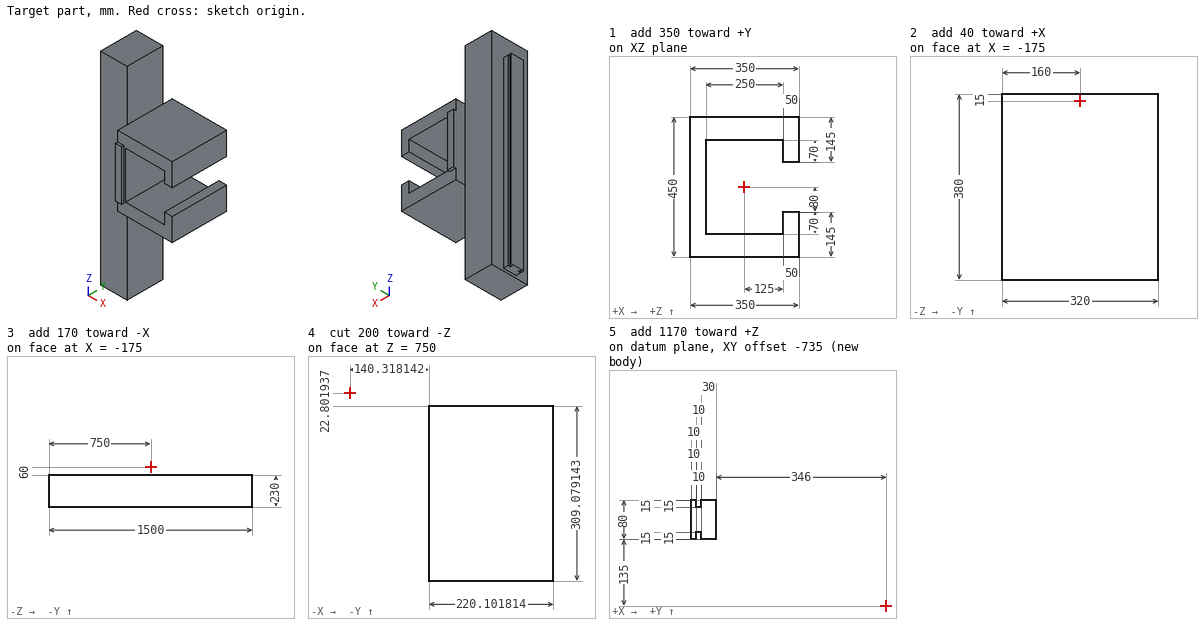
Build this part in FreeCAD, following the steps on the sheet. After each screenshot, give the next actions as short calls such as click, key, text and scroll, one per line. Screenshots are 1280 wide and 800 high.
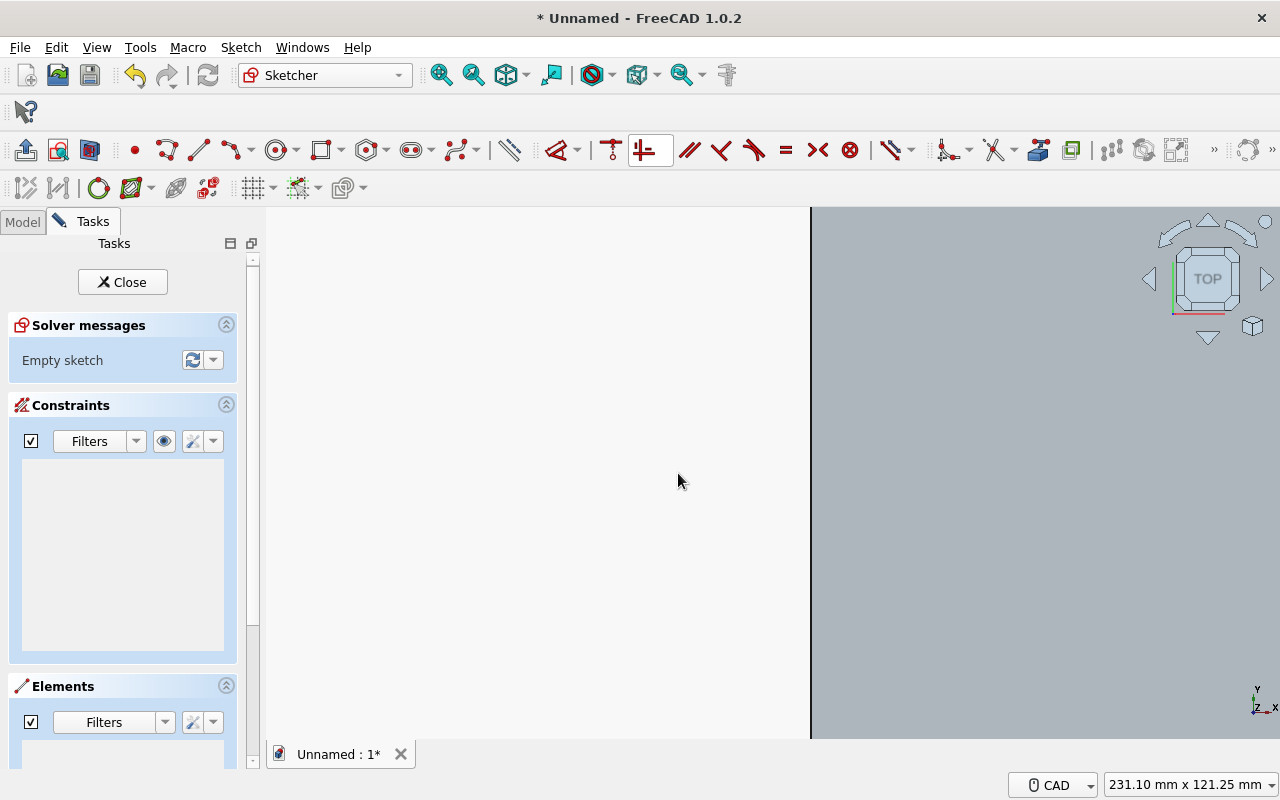
key(g)
key(m)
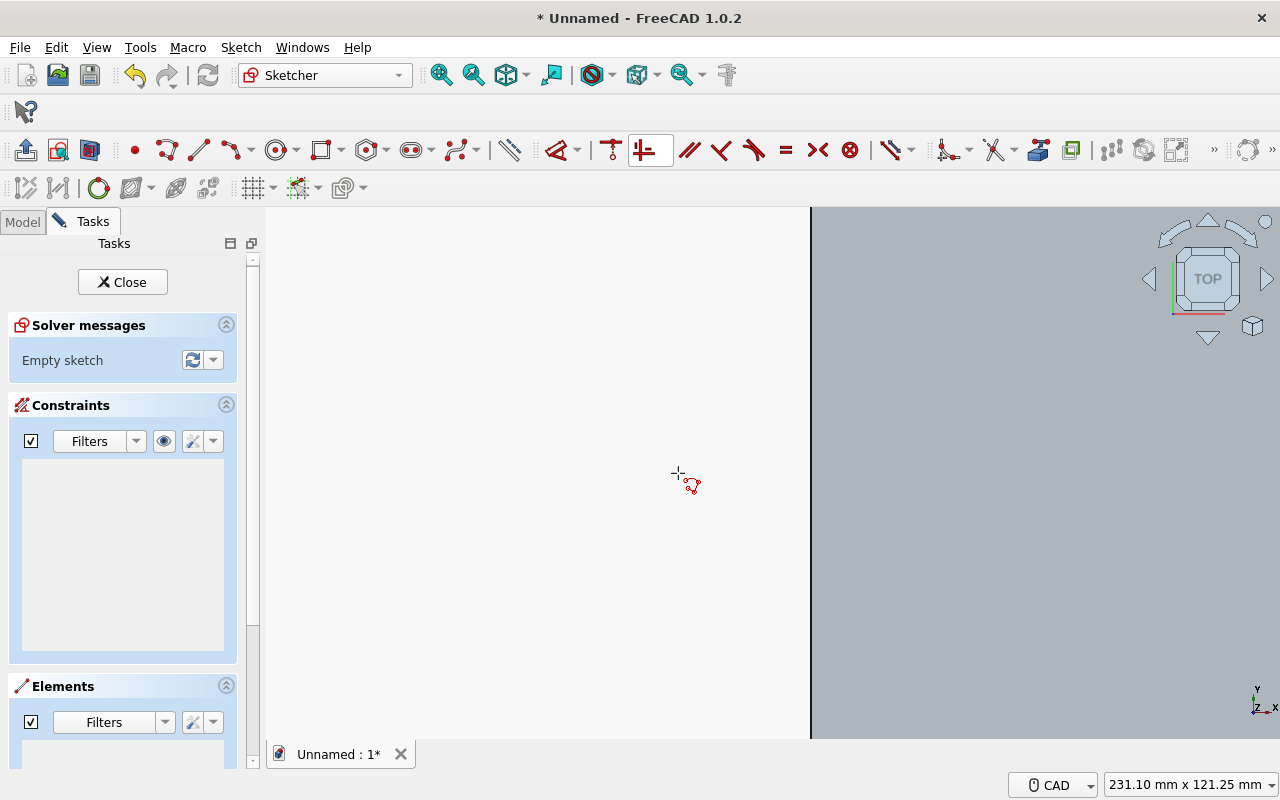
click(807, 642)
click(675, 642)
click(675, 576)
click(631, 576)
click(631, 642)
click(587, 642)
click(587, 291)
click(631, 291)
click(631, 357)
click(675, 357)
click(675, 291)
click(807, 291)
click(807, 643)
key(Escape)
key(Escape)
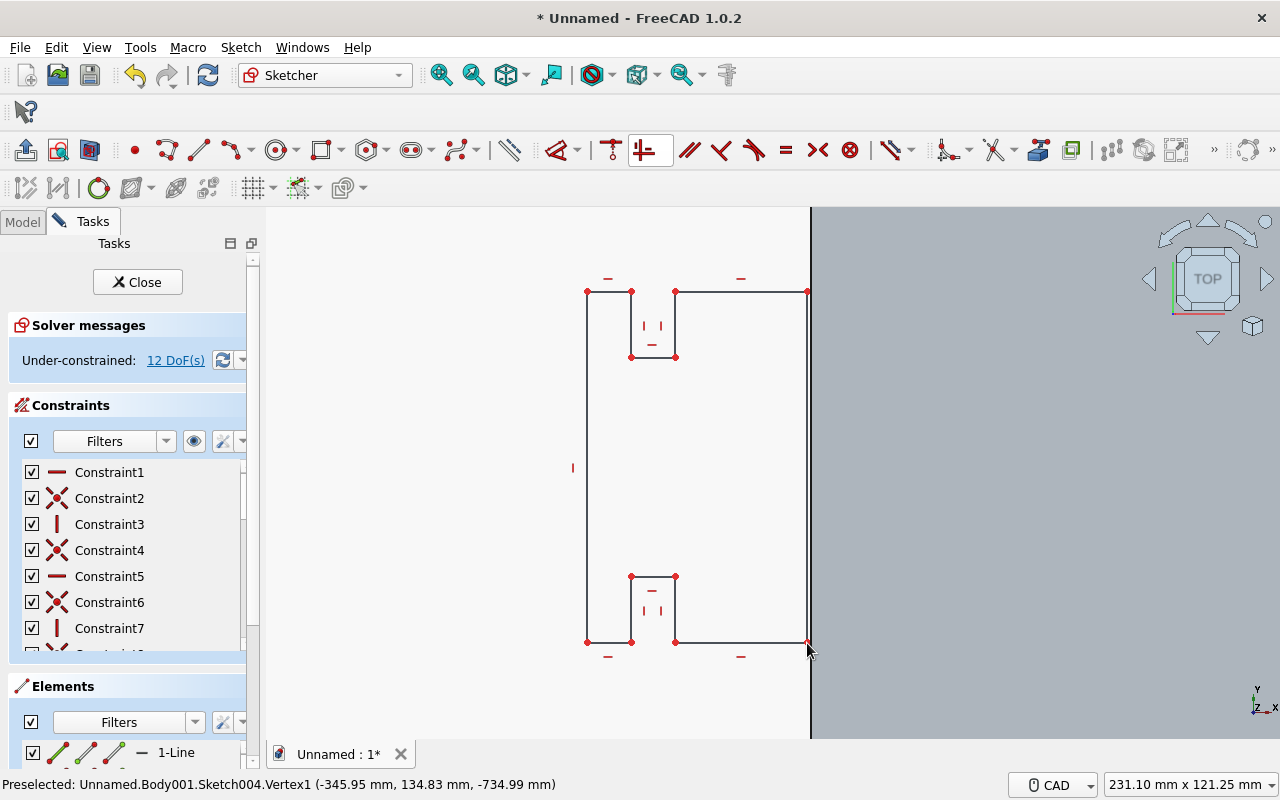
click(556, 150)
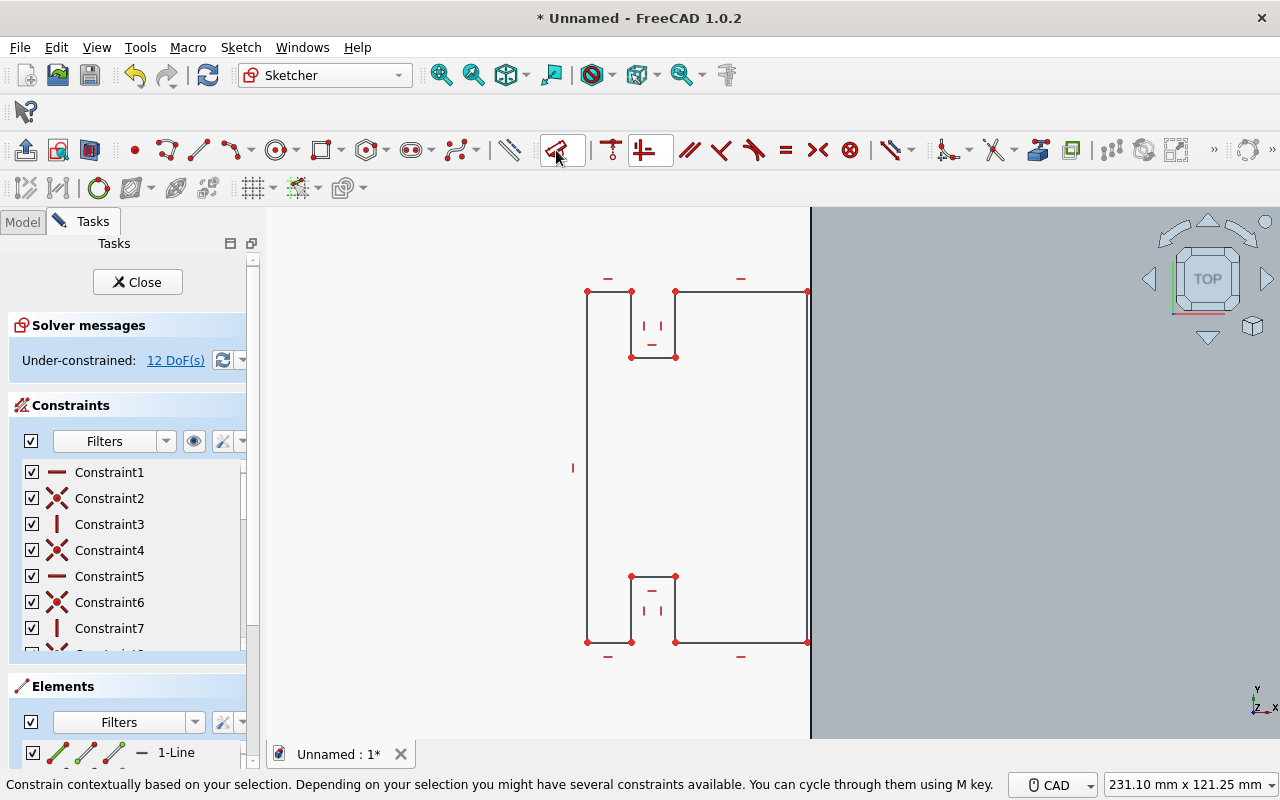
click(767, 643)
click(741, 677)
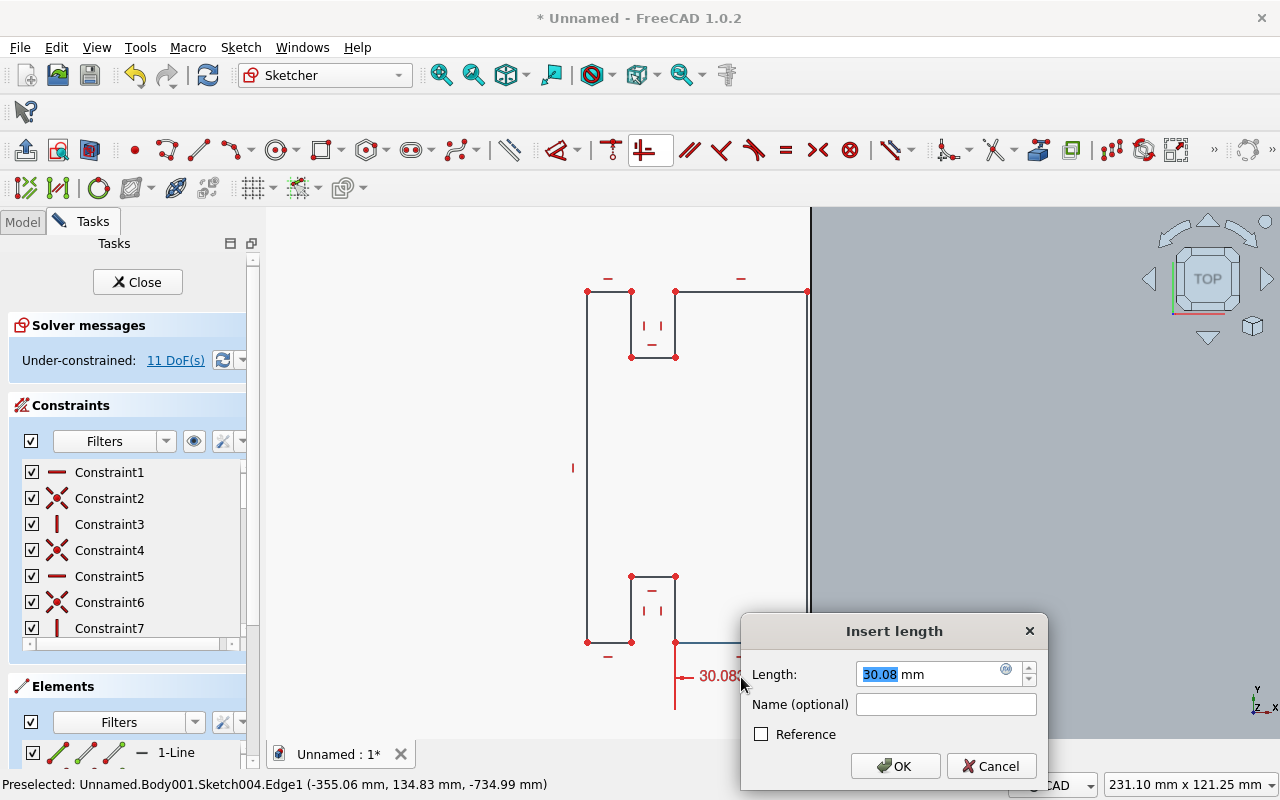
text(30)
key(Return)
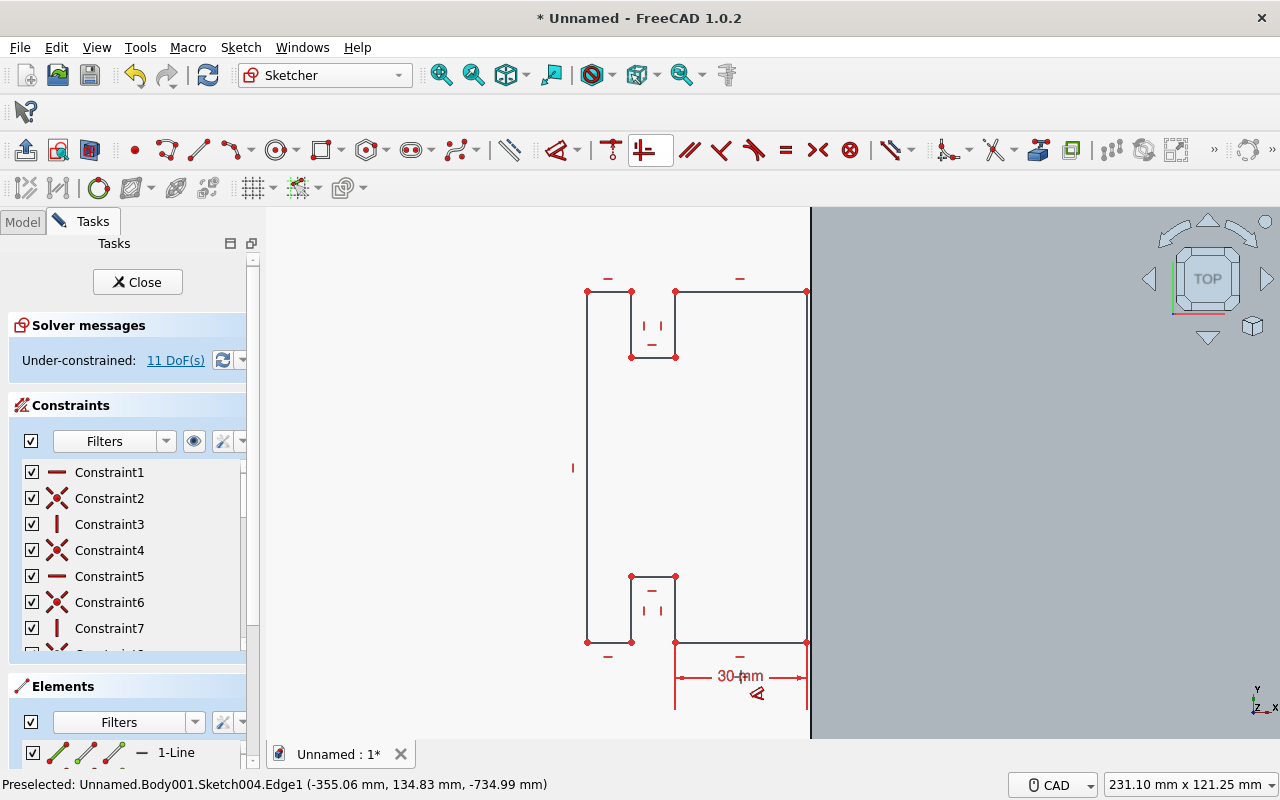
click(675, 623)
click(709, 610)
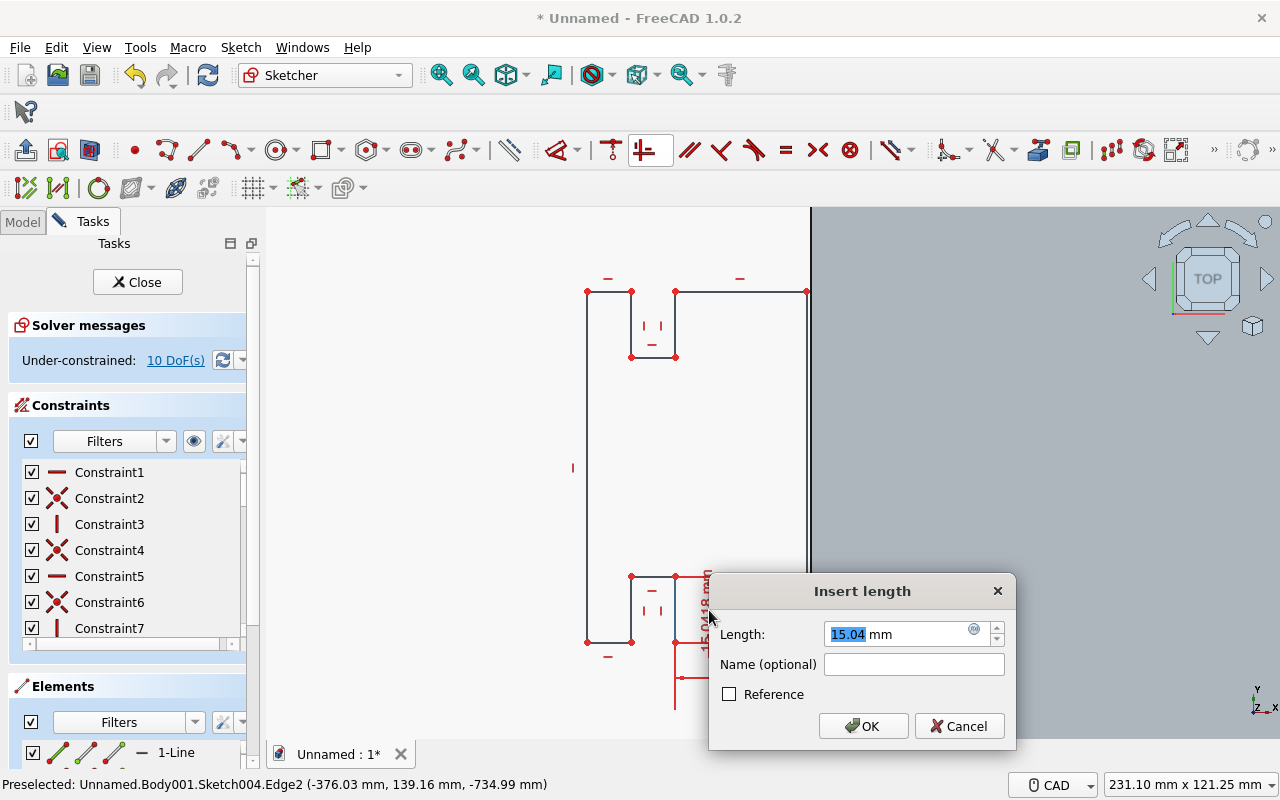
text(15)
key(Return)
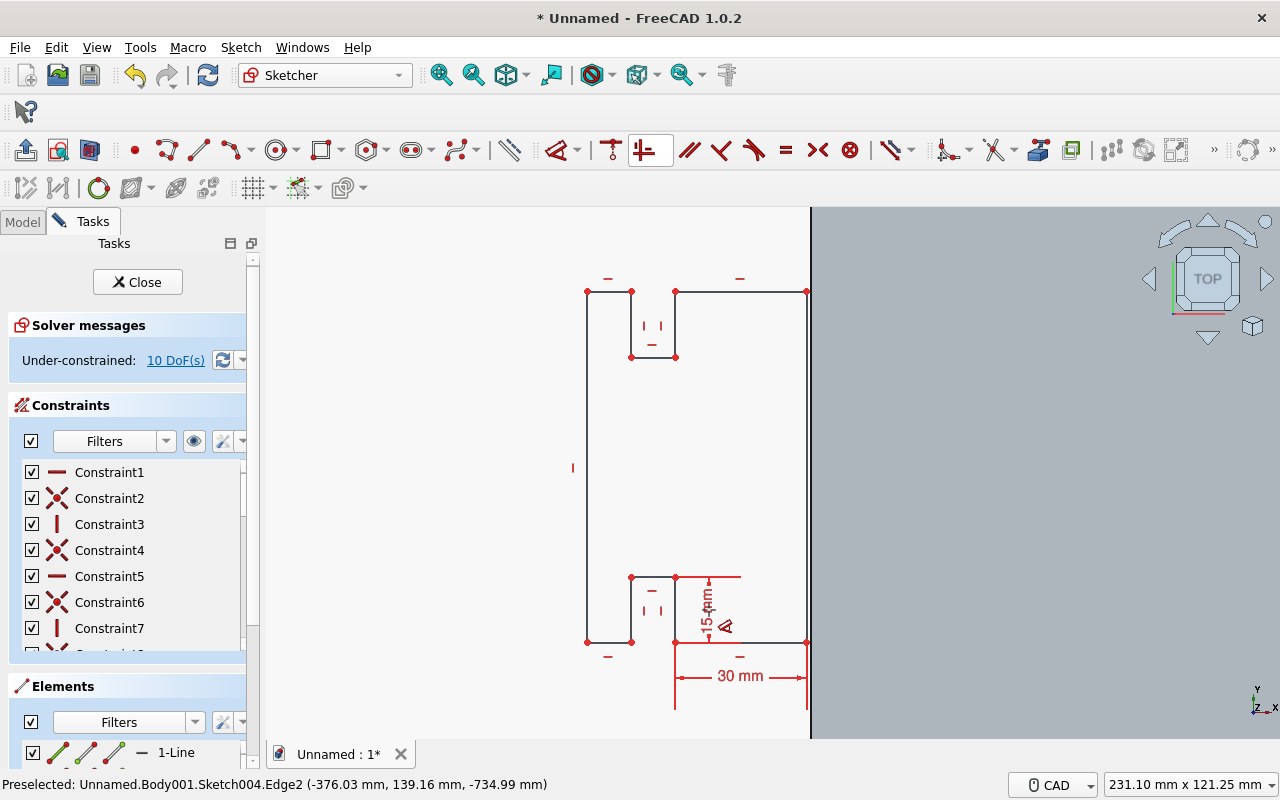
click(662, 577)
click(653, 543)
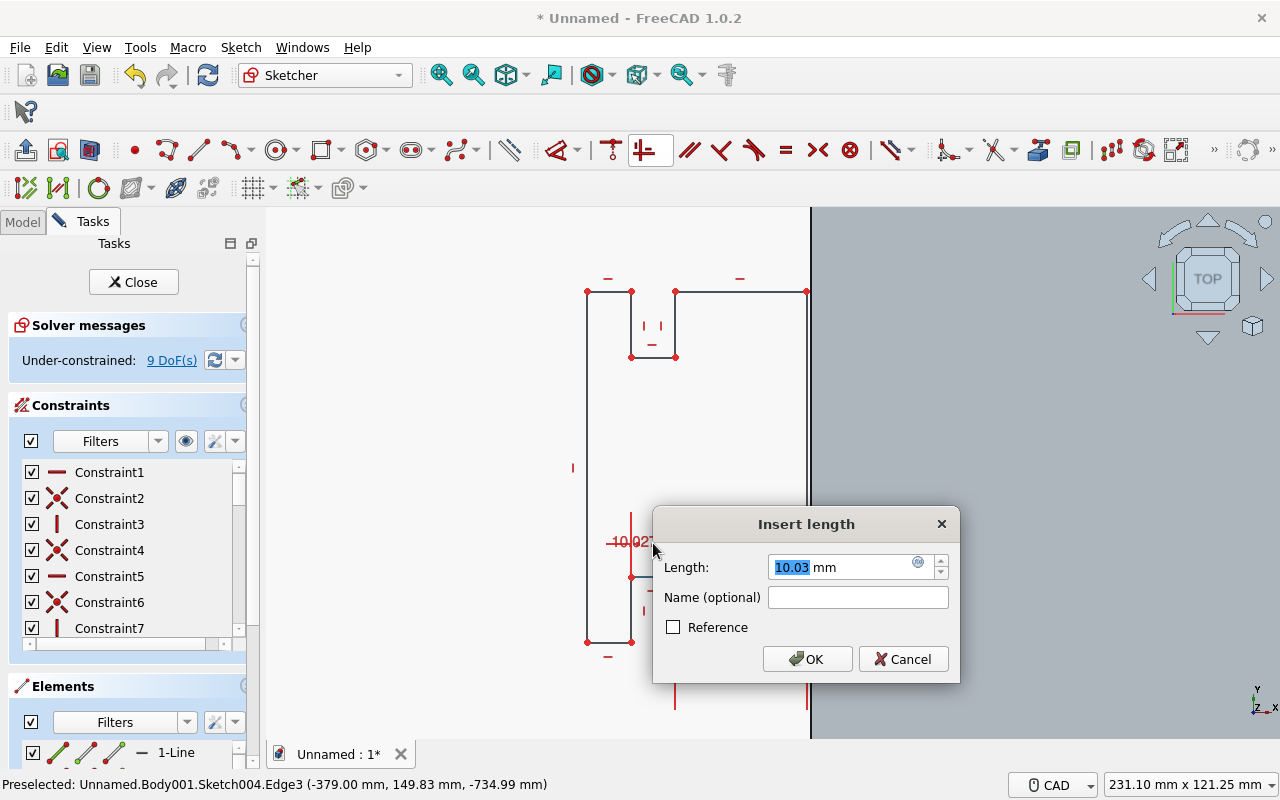
text(10)
key(Return)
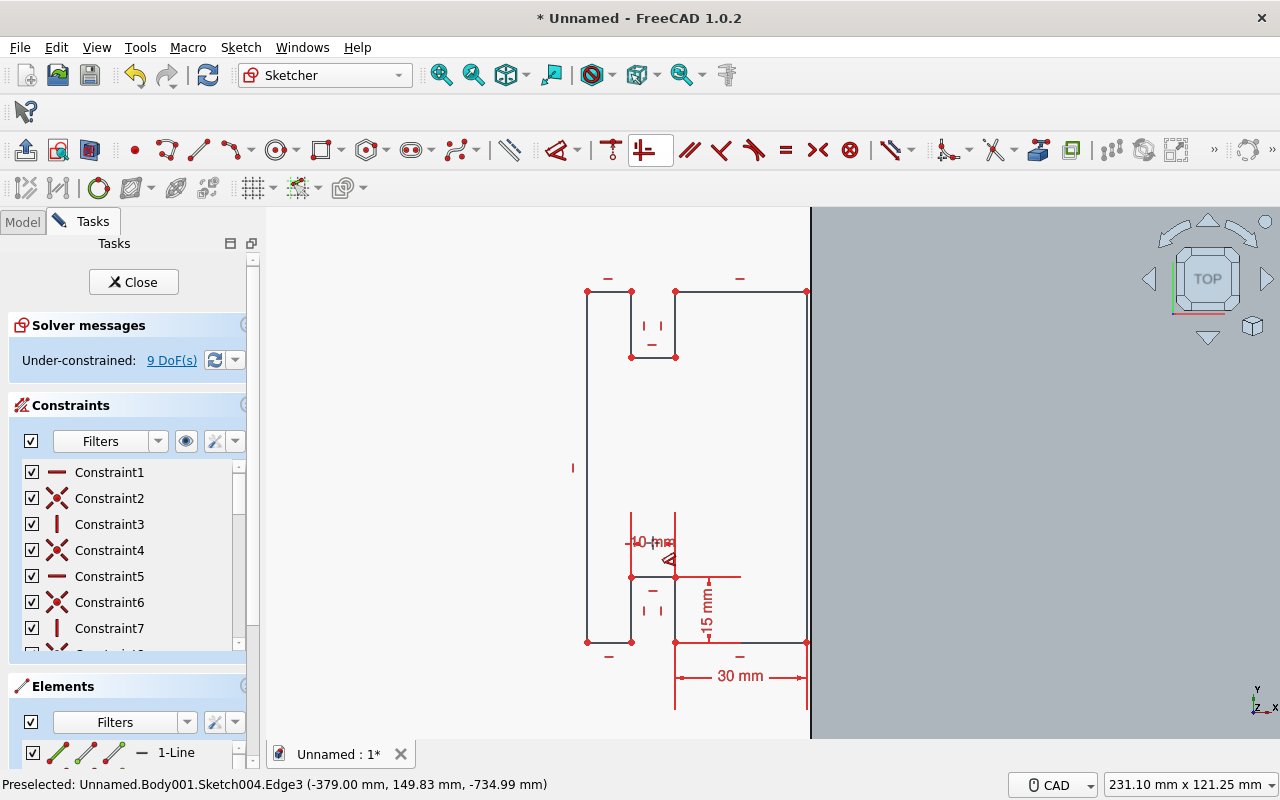
click(631, 597)
click(573, 610)